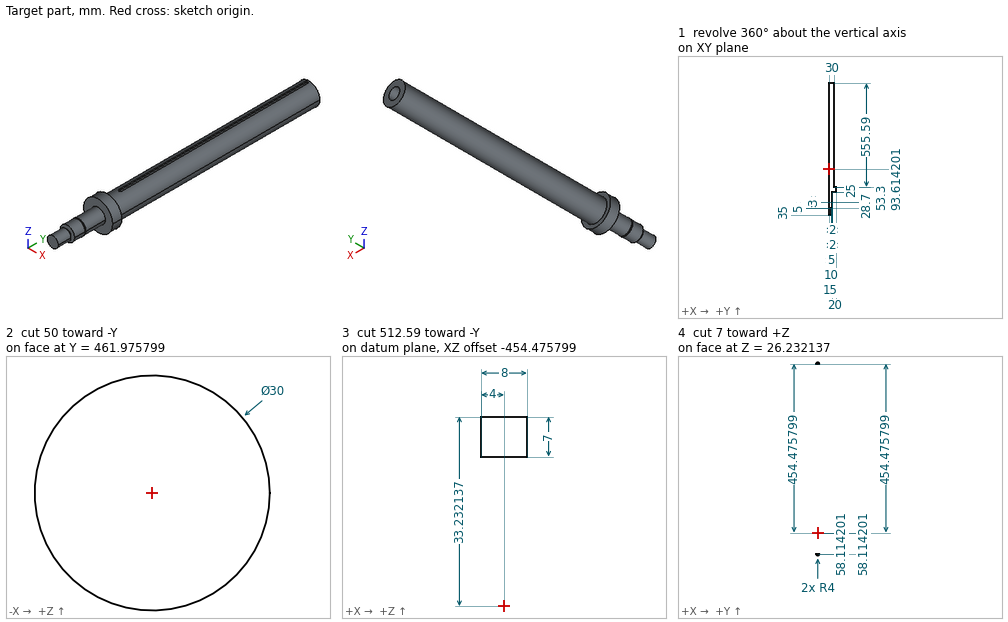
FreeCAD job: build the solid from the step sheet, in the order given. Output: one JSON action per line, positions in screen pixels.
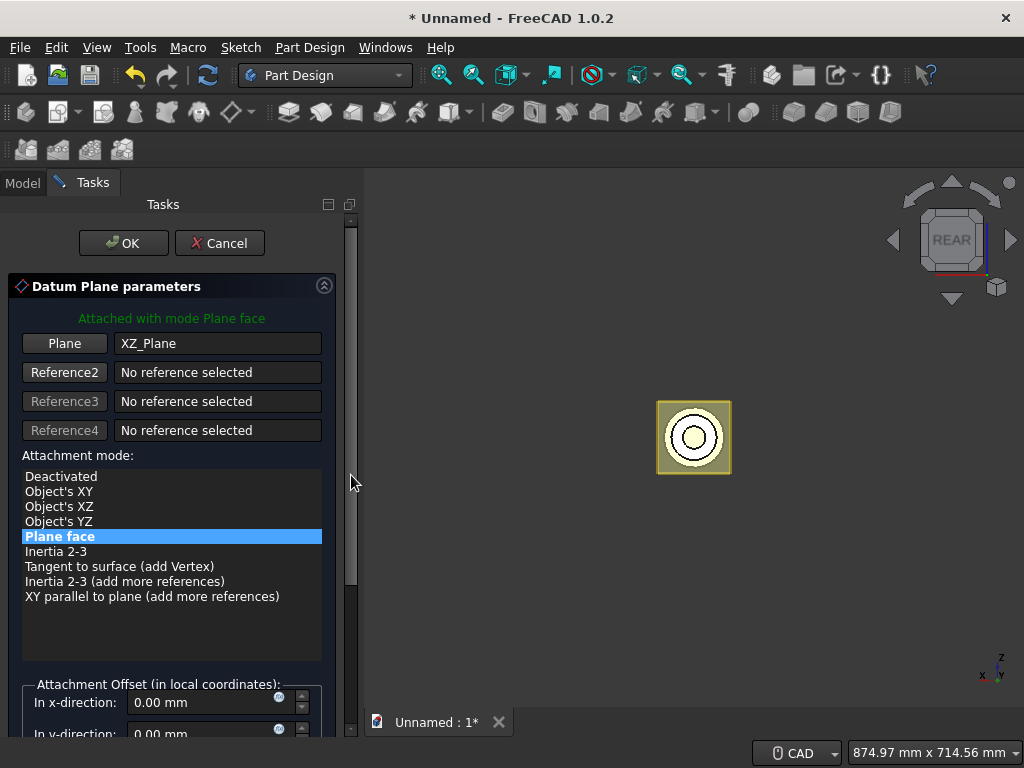
{"action": "left_click", "coordinate": [124, 243]}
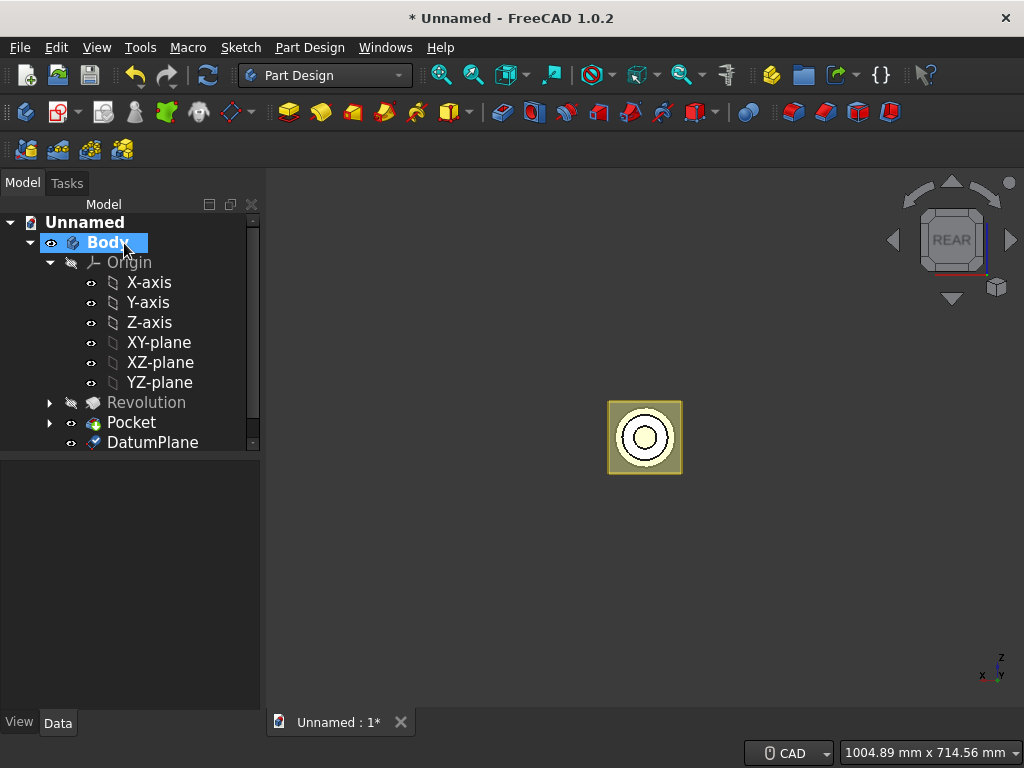
{"action": "left_click", "coordinate": [116, 443]}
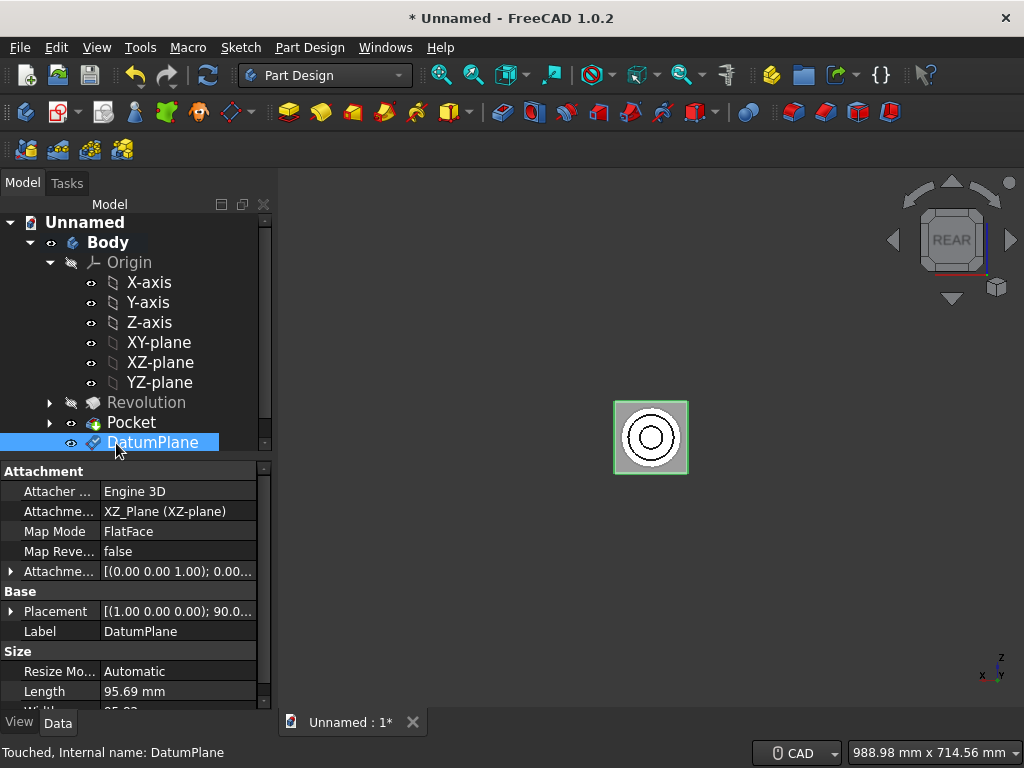
{"action": "left_click", "coordinate": [58, 112]}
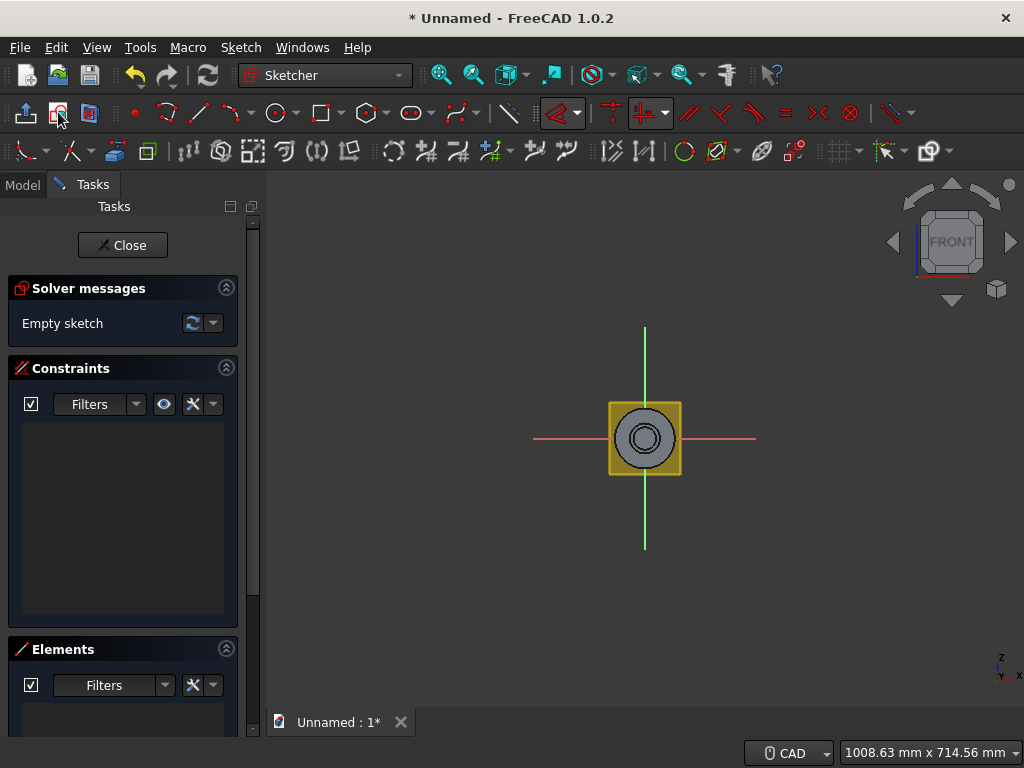
{"action": "left_click", "coordinate": [90, 114]}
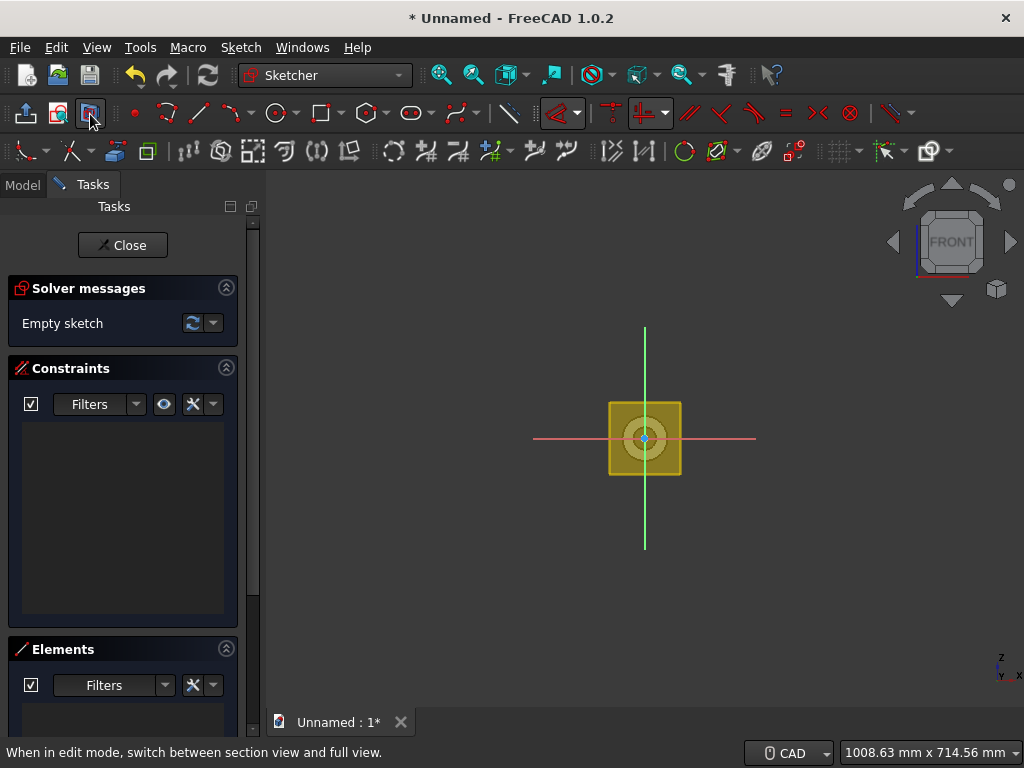
{"action": "scroll", "coordinate": [648, 415], "scroll_direction": "up", "scroll_amount": 15}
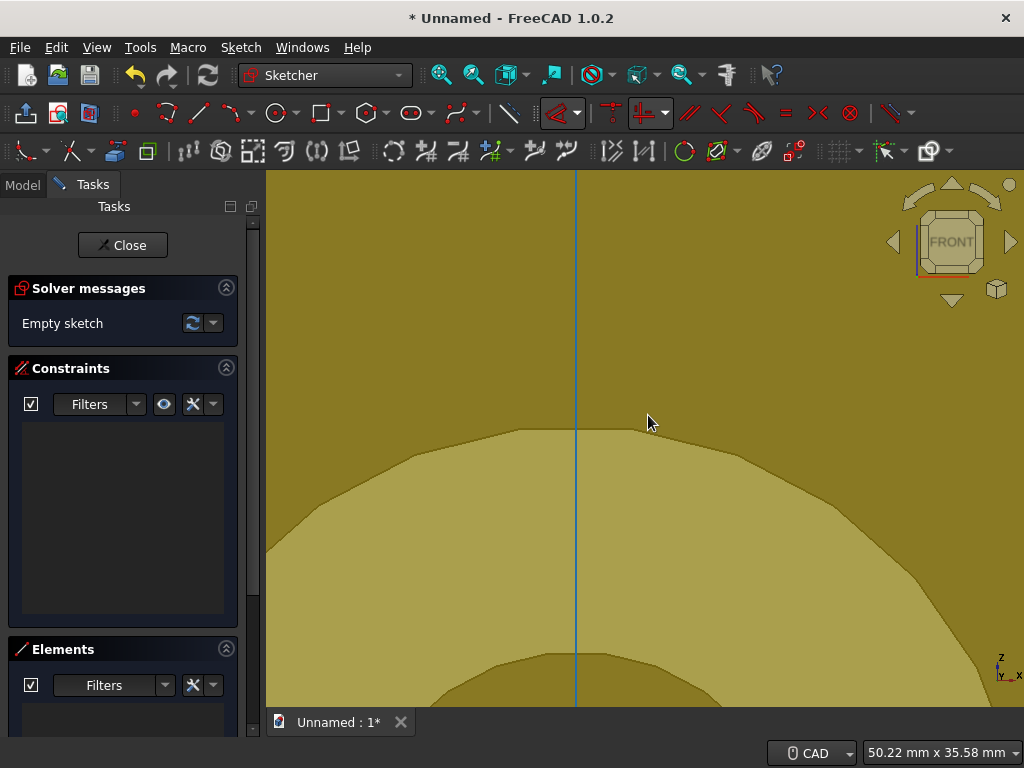
{"action": "scroll", "coordinate": [576, 426], "scroll_direction": "up", "scroll_amount": 6}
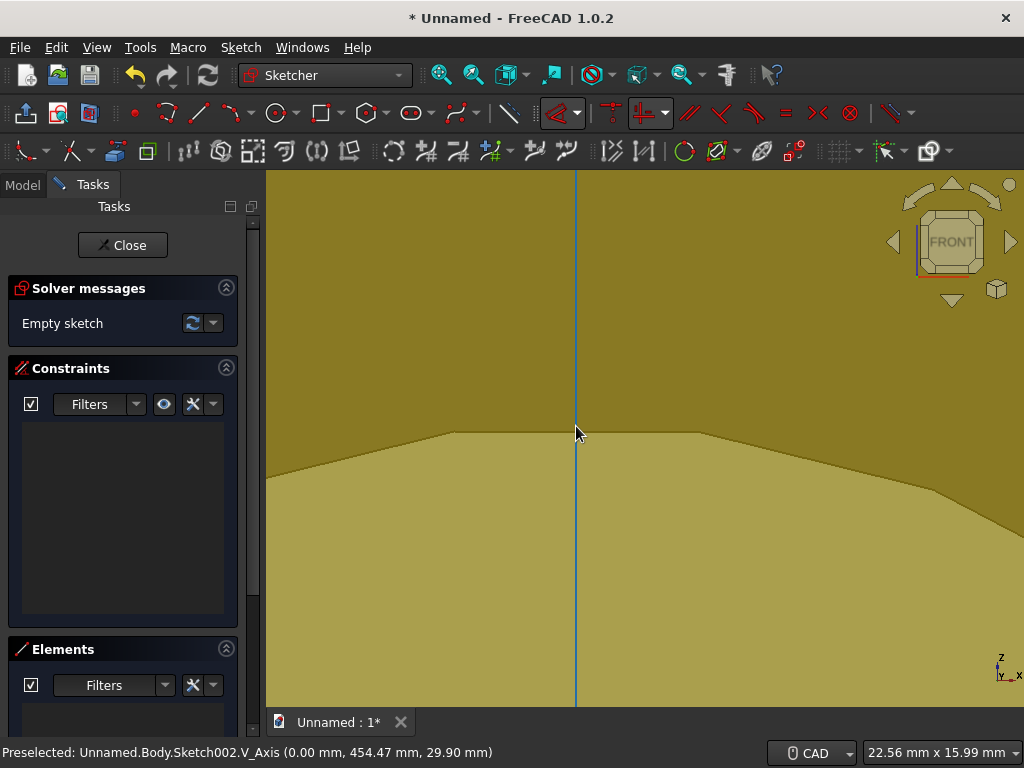
{"action": "key", "text": "g r"}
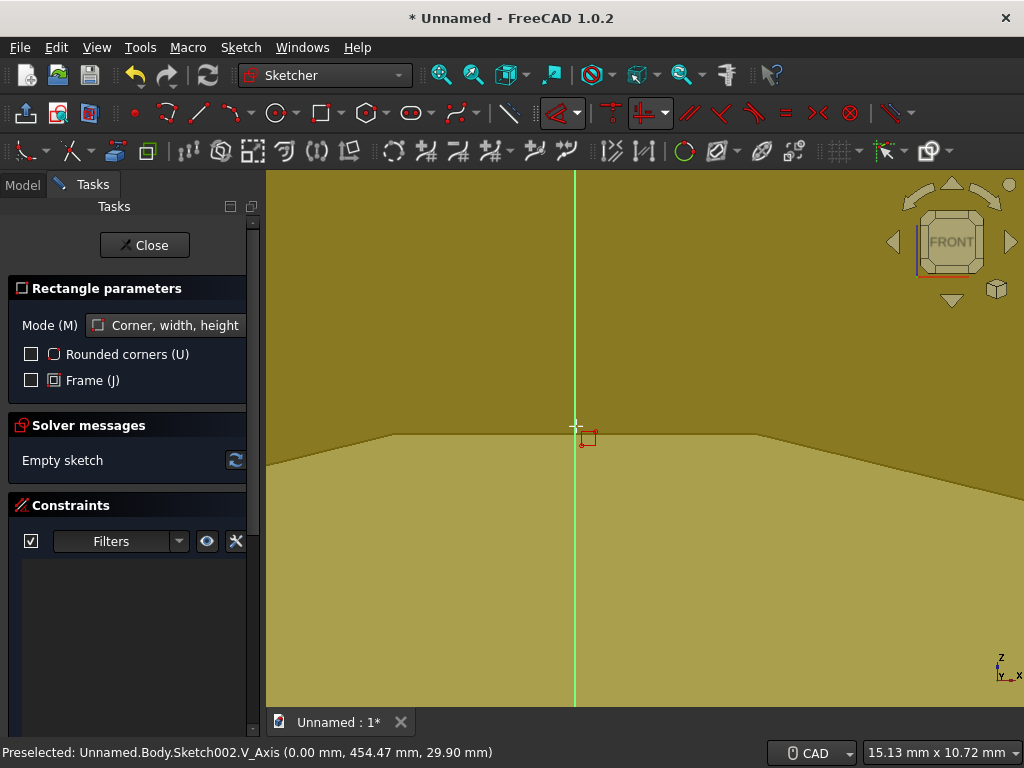
{"action": "left_click", "coordinate": [375, 261]}
{"action": "mouse_move", "coordinate": [776, 612]}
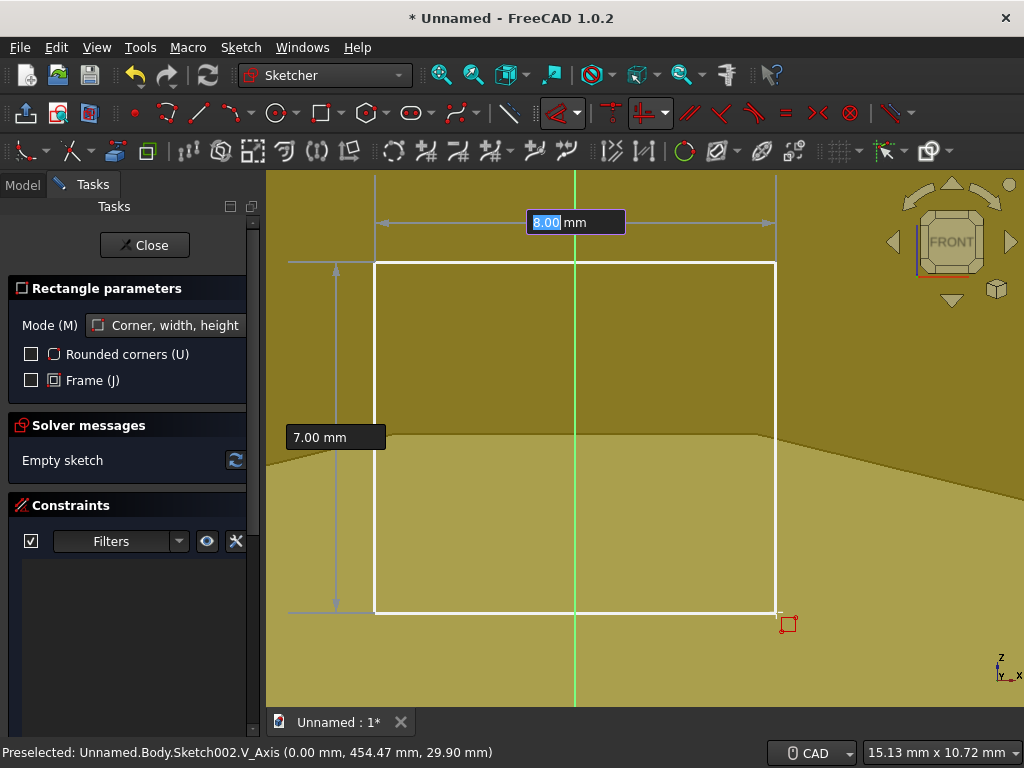
{"action": "type", "text": "8"}
{"action": "key", "text": "Tab"}
{"action": "type", "text": "7"}
{"action": "key", "text": "Return"}
{"action": "key", "text": "Escape"}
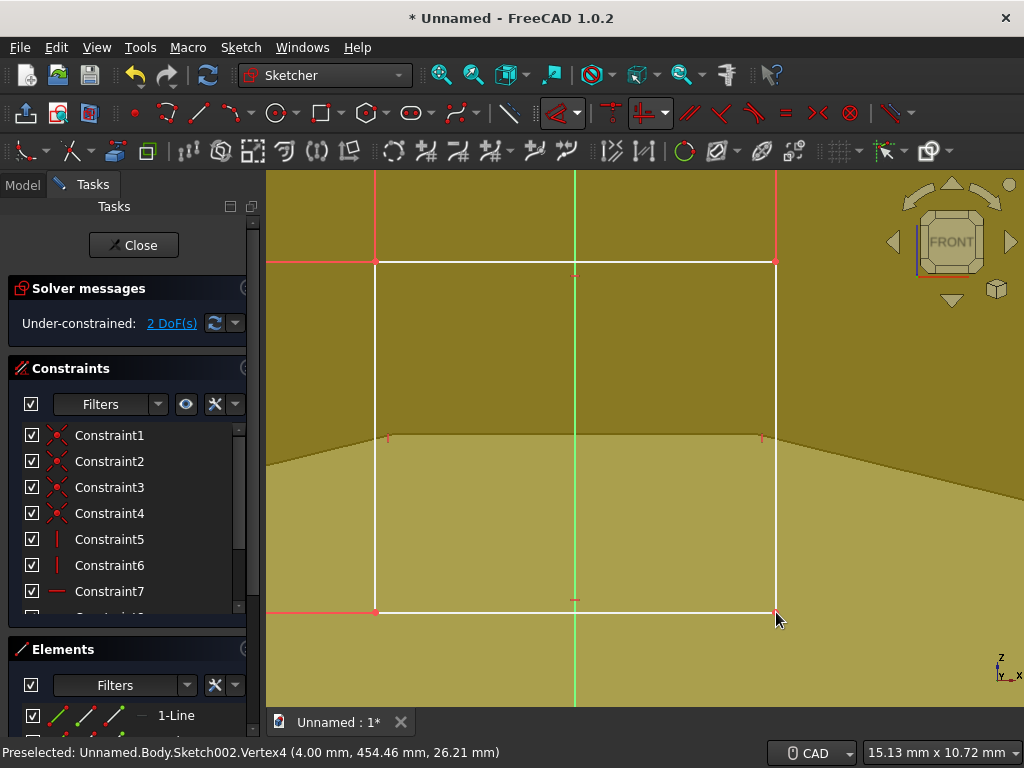
{"action": "key", "text": "d"}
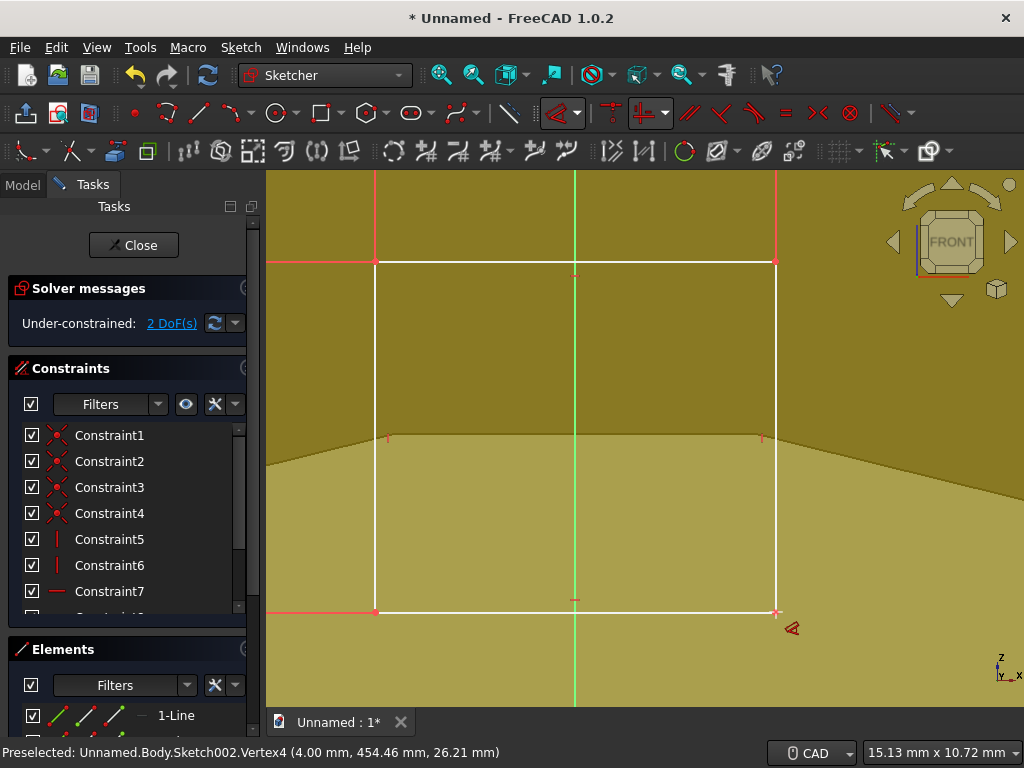
{"action": "left_click", "coordinate": [375, 262]}
{"action": "left_click", "coordinate": [475, 228]}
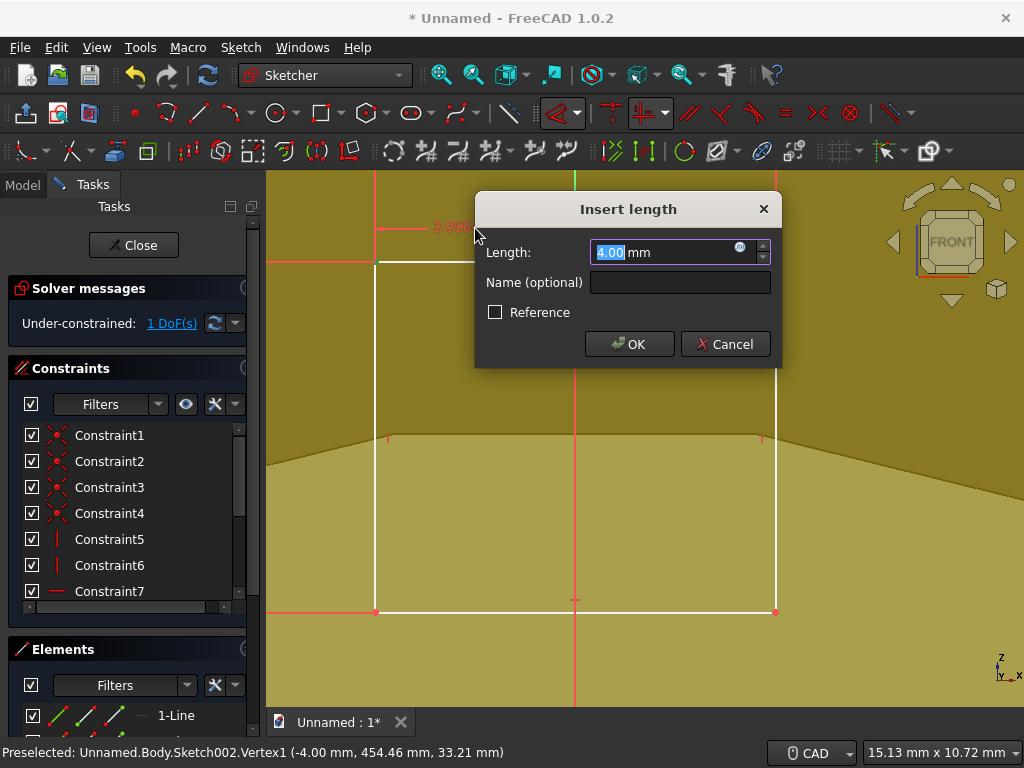
{"action": "type", "text": "4"}
{"action": "key", "text": "Return"}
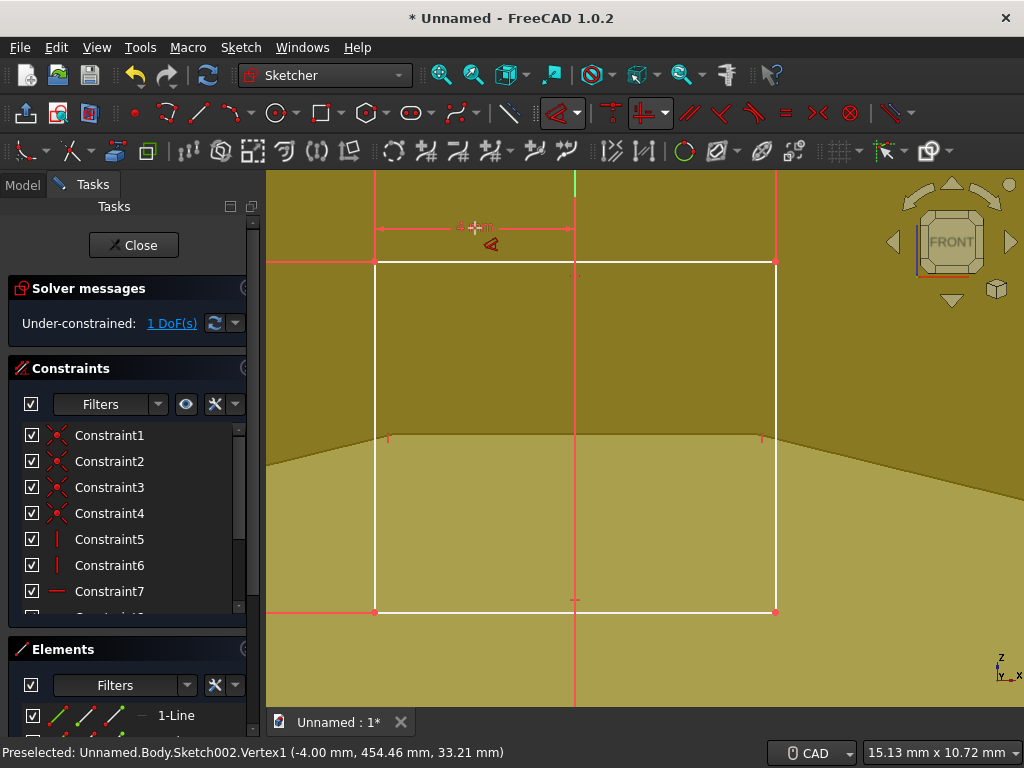
{"action": "left_click", "coordinate": [375, 262]}
{"action": "left_click", "coordinate": [341, 471]}